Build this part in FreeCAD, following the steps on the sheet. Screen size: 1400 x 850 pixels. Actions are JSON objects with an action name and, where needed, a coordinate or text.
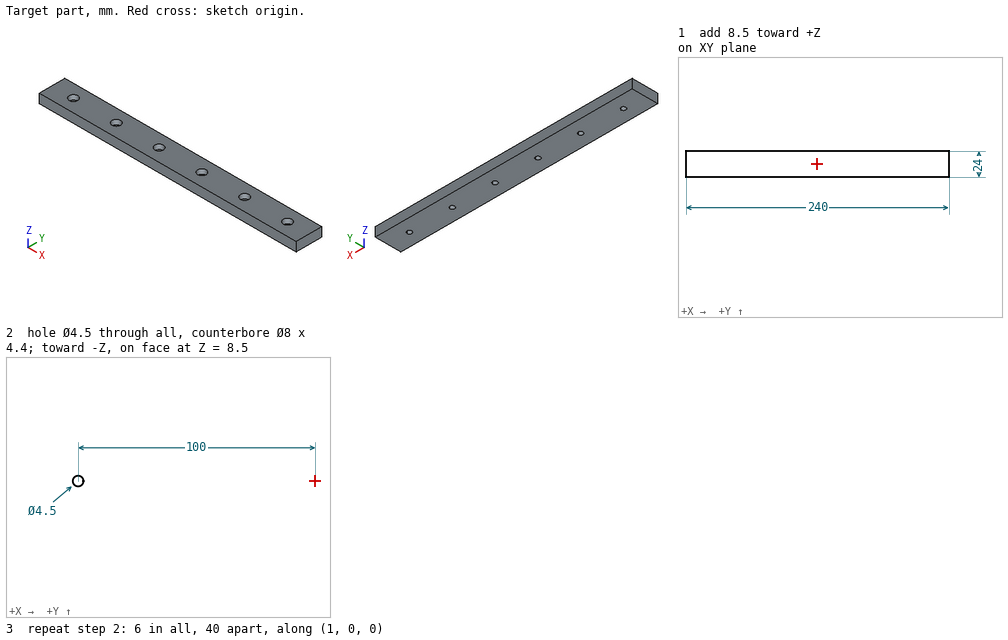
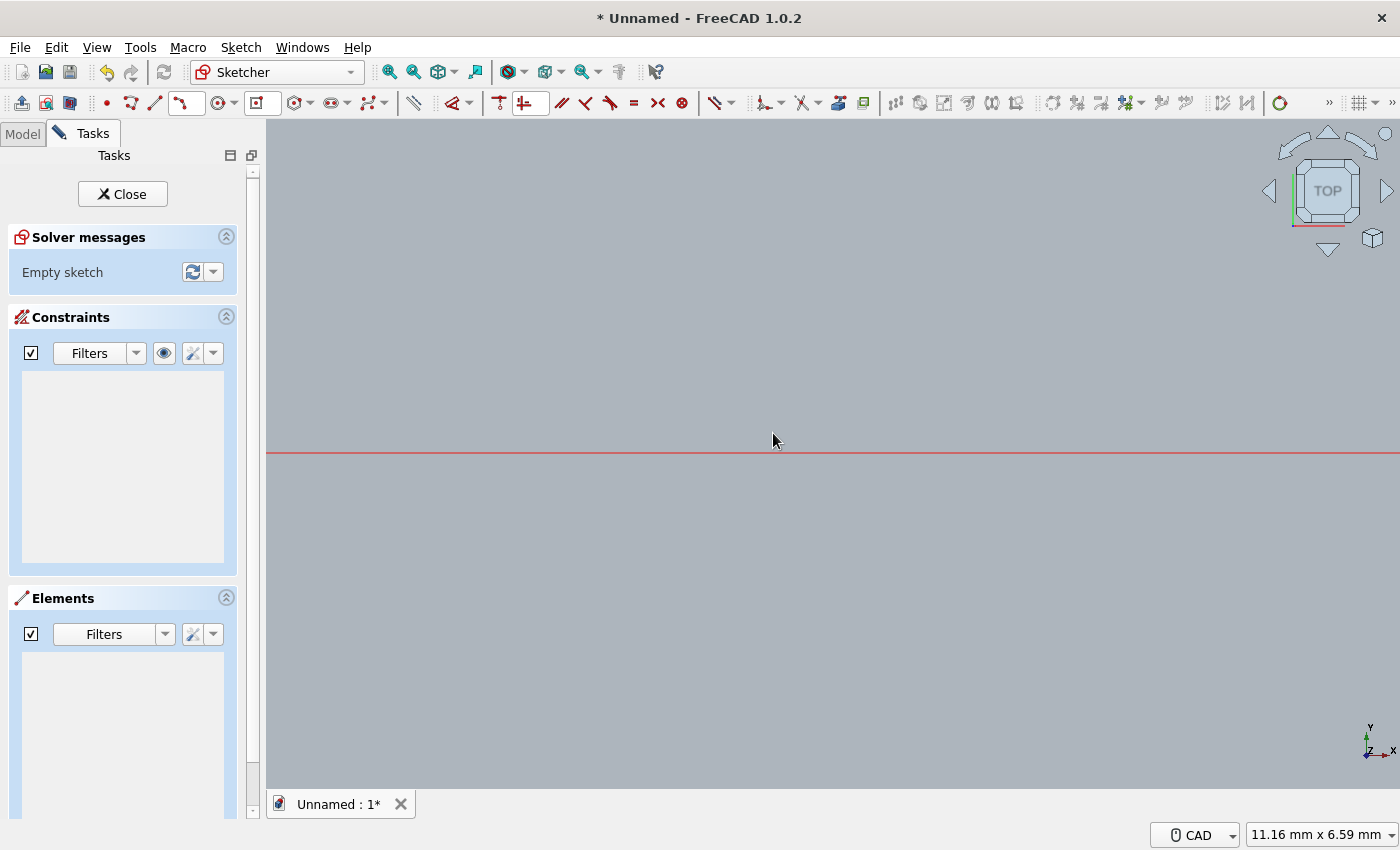
{"action": "key", "text": "g c"}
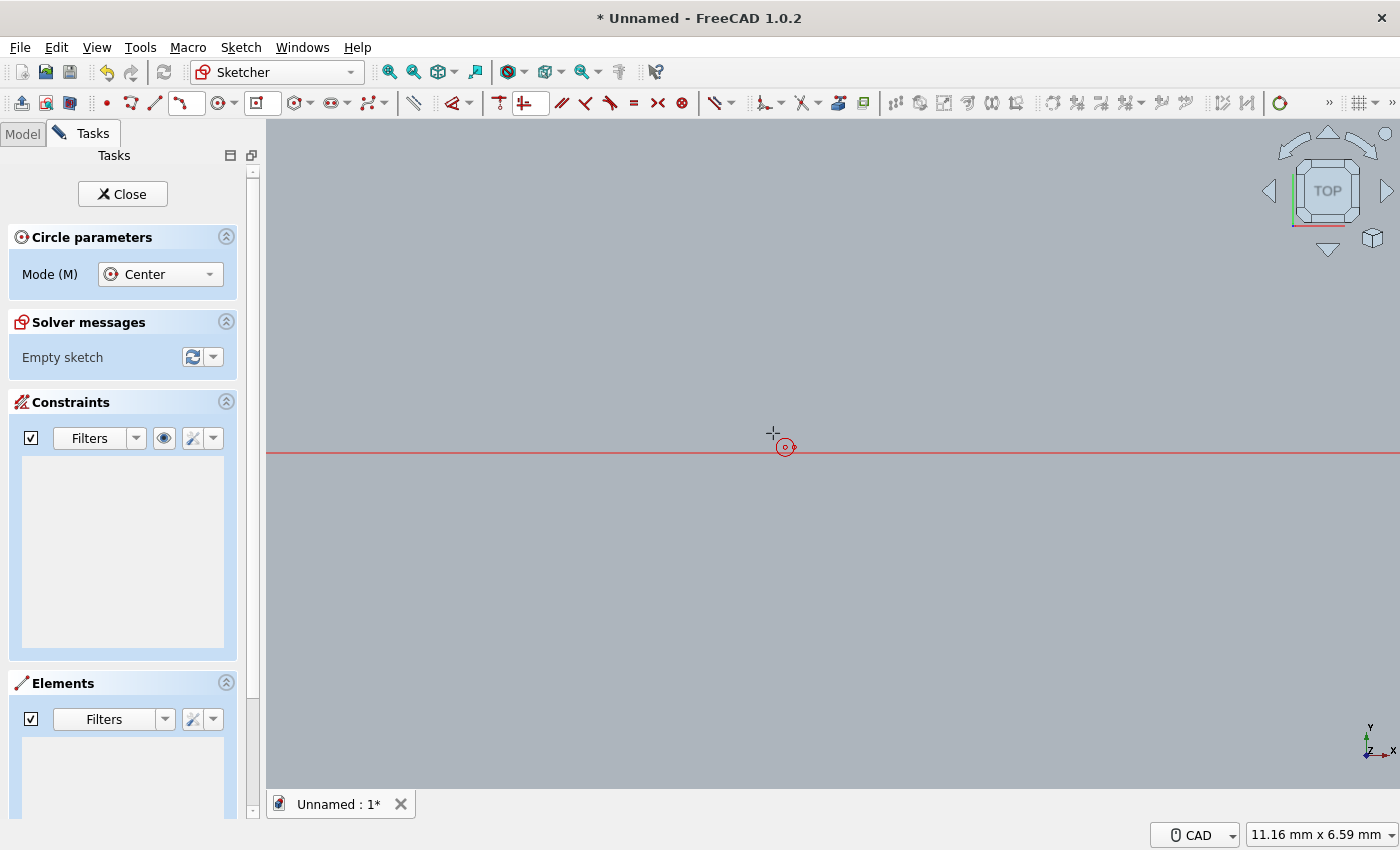
{"action": "left_click", "coordinate": [764, 453]}
{"action": "mouse_move", "coordinate": [925, 292]}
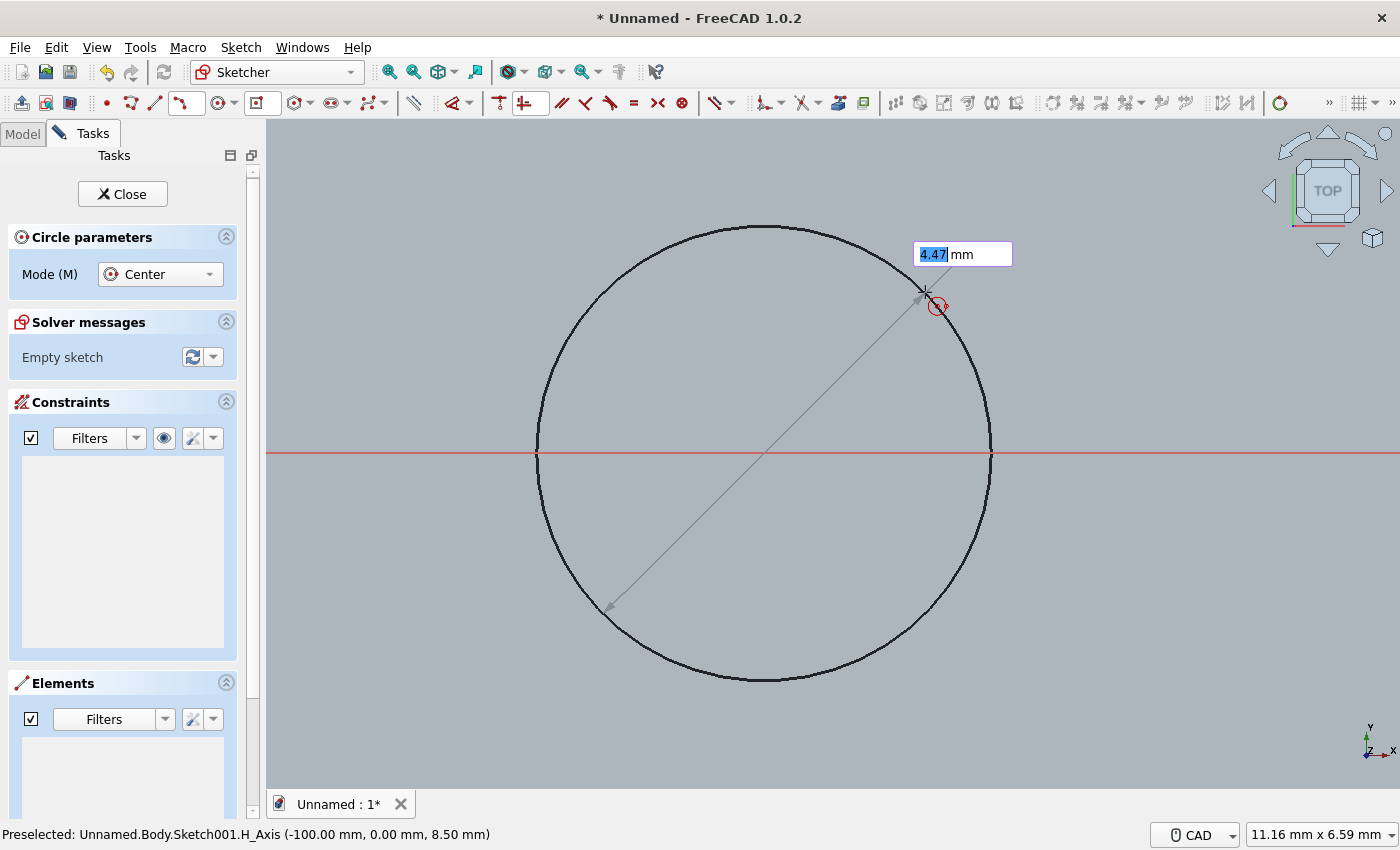
{"action": "type", "text": "4.5"}
{"action": "key", "text": "Return"}
{"action": "key", "text": "Escape"}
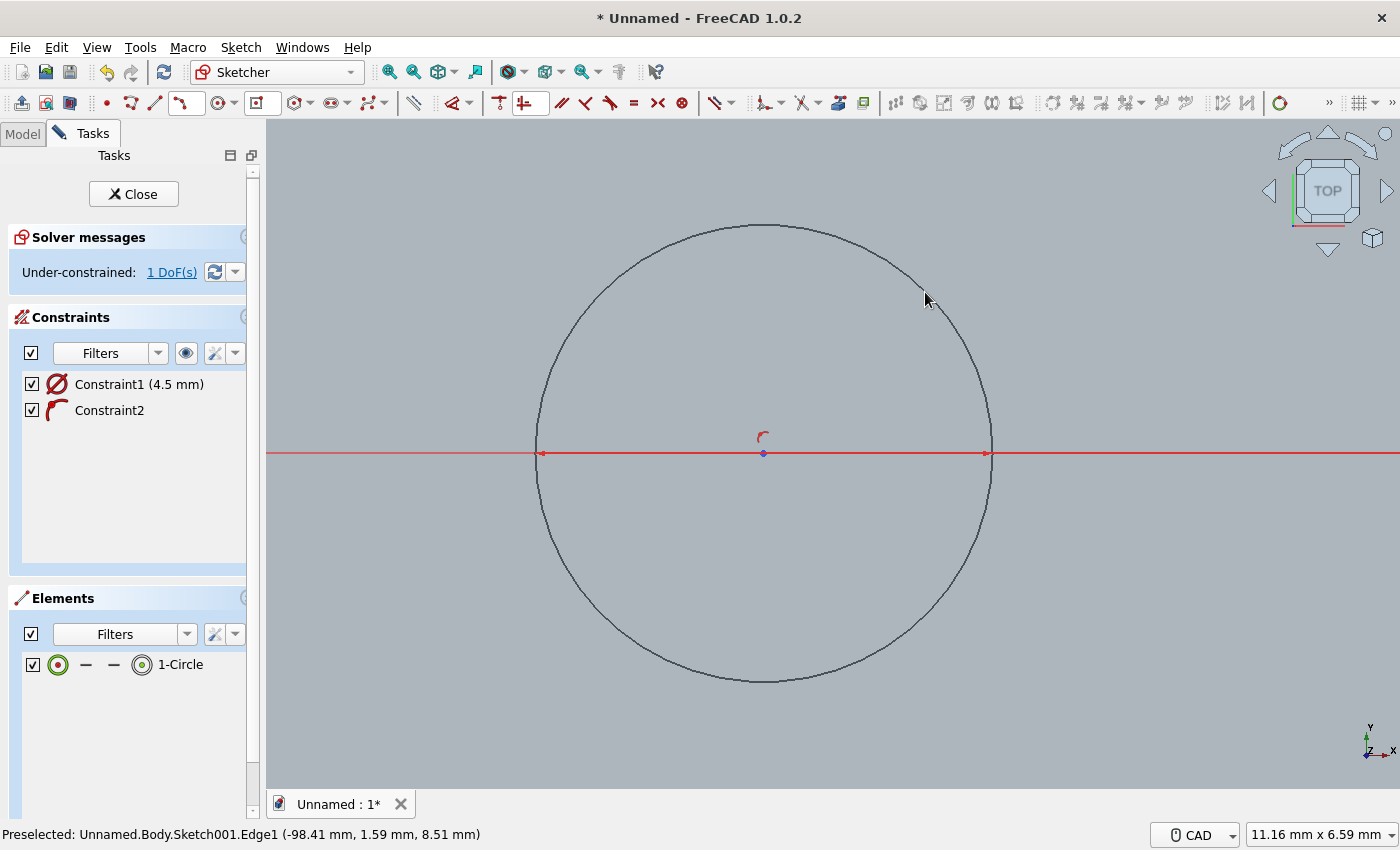
{"action": "key", "text": "d"}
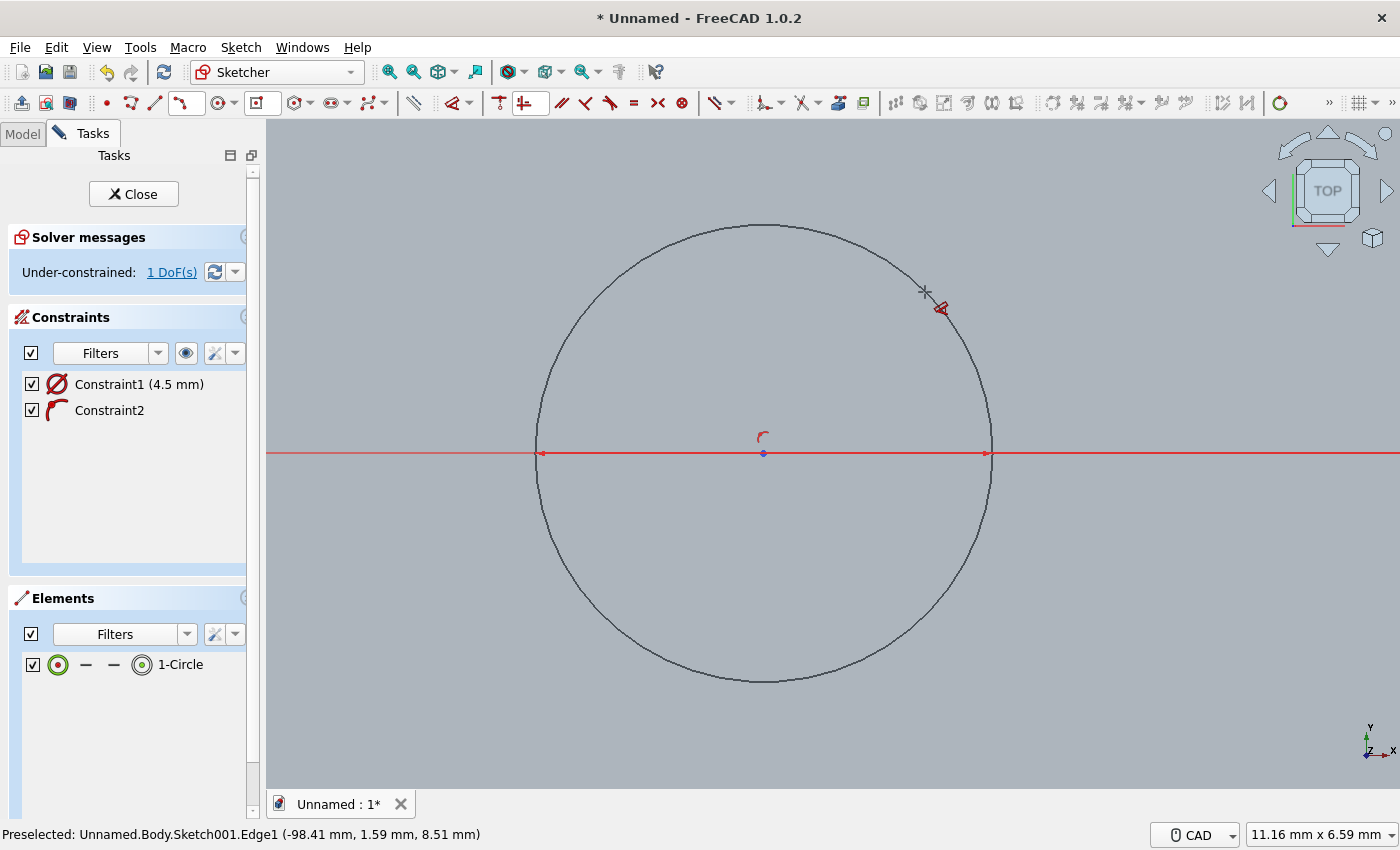
{"action": "left_click", "coordinate": [764, 453]}
{"action": "left_click", "coordinate": [891, 487]}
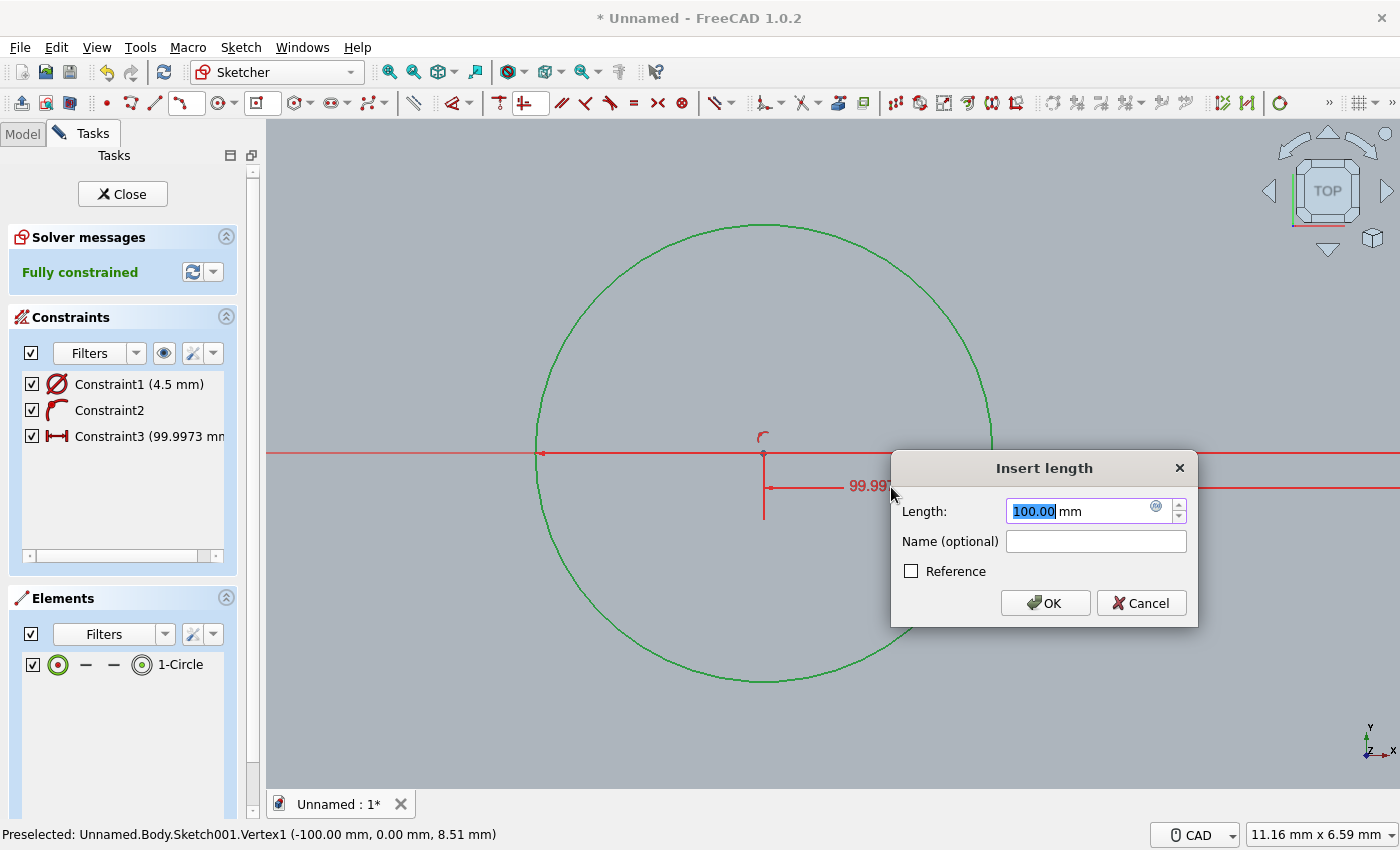
{"action": "type", "text": "100"}
{"action": "key", "text": "Return"}
{"action": "key", "text": "Escape"}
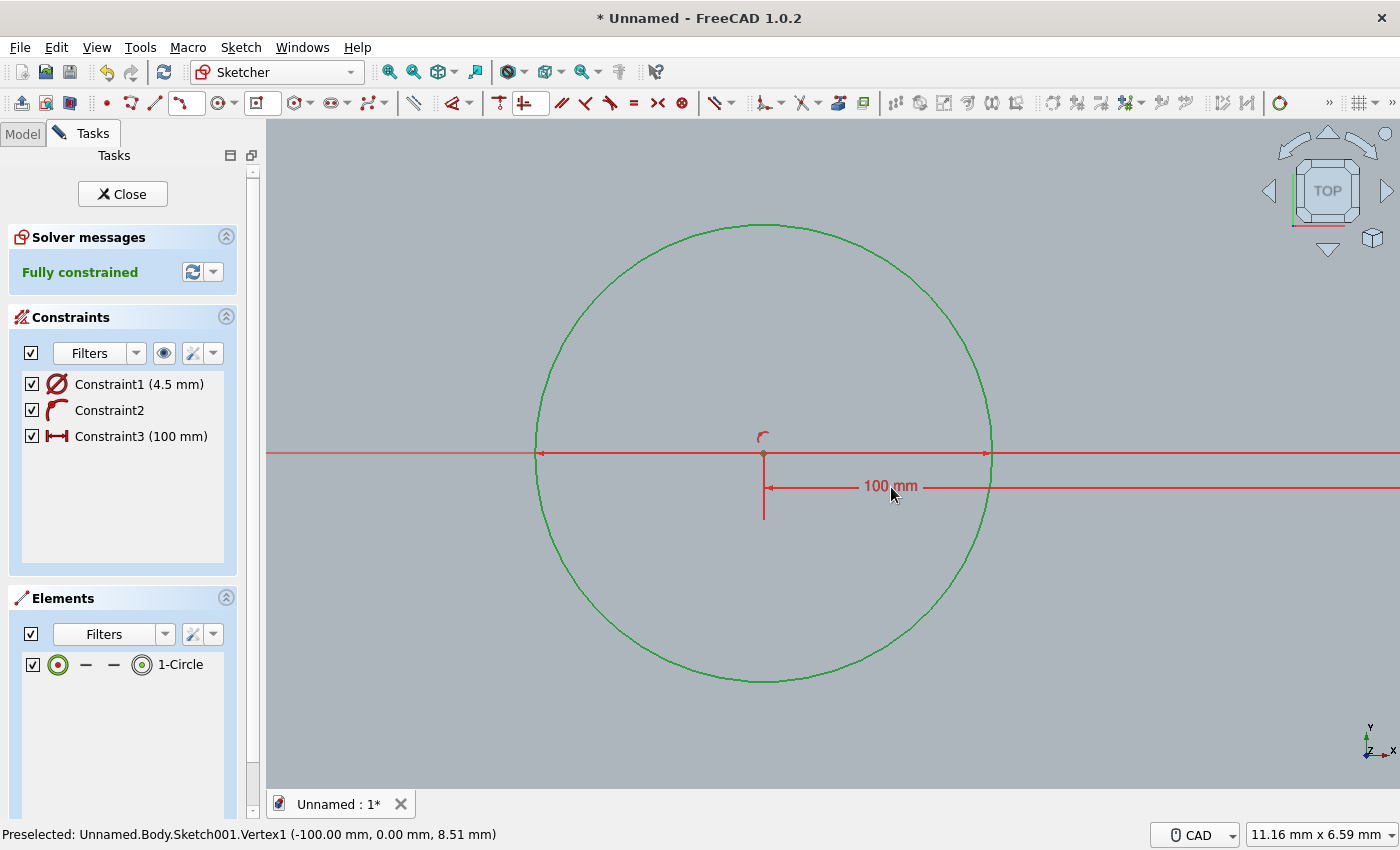
{"action": "left_click", "coordinate": [123, 194]}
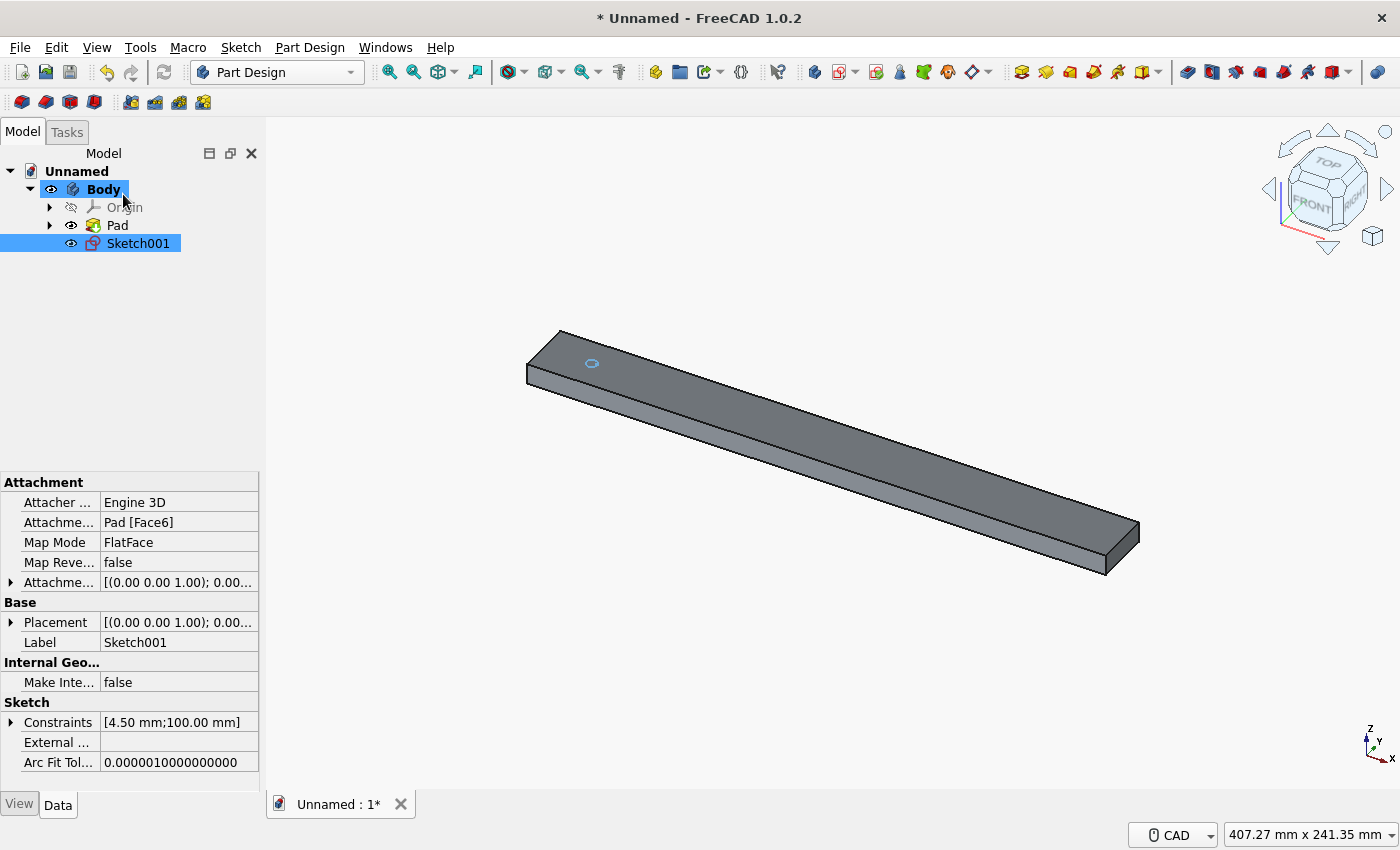
{"action": "left_click", "coordinate": [1212, 72]}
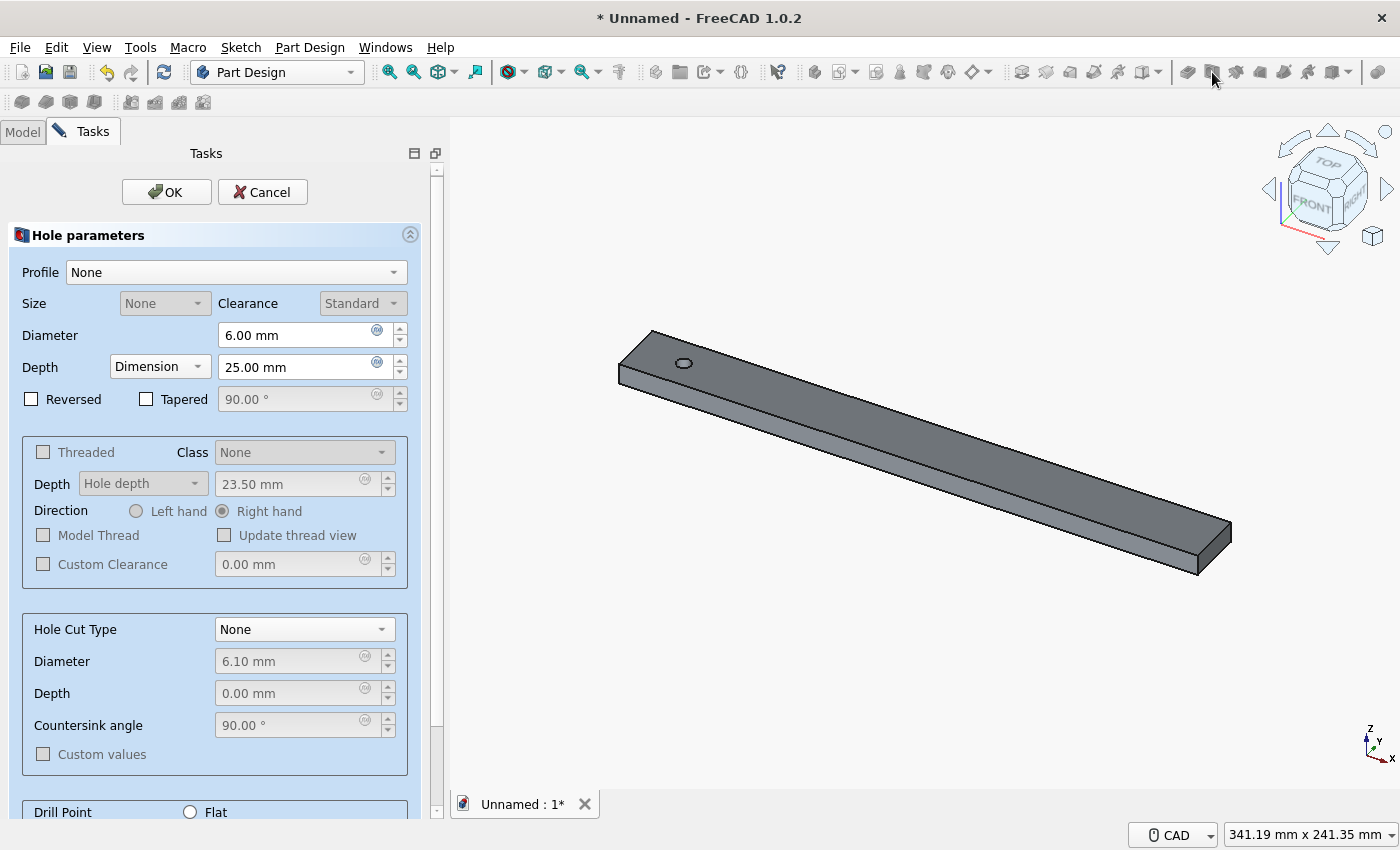
{"action": "triple_click", "coordinate": [305, 335]}